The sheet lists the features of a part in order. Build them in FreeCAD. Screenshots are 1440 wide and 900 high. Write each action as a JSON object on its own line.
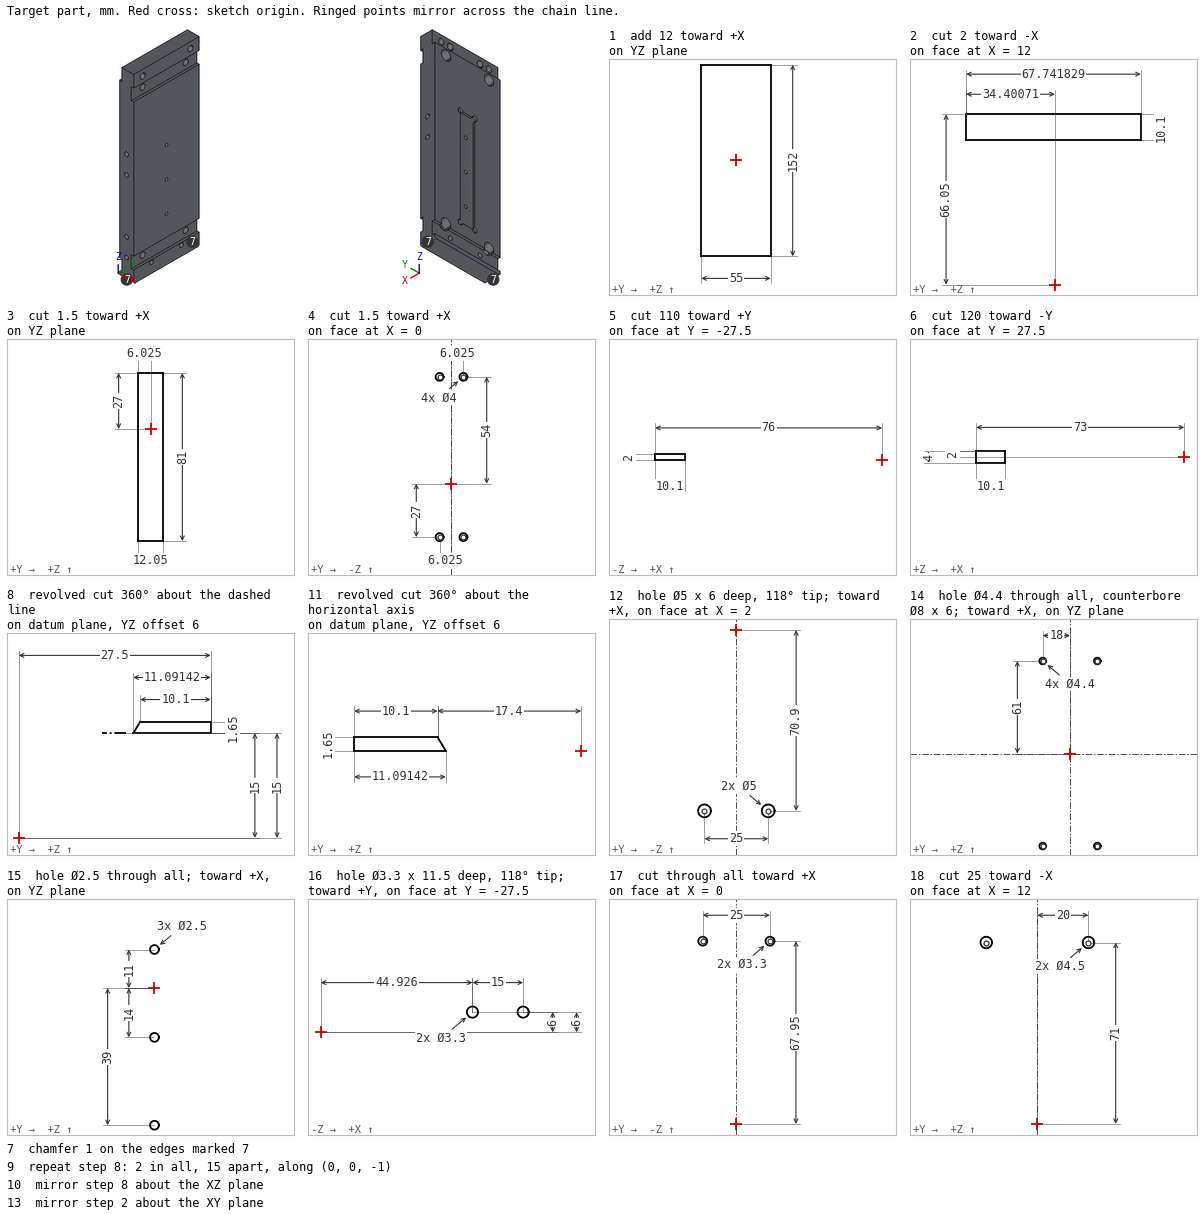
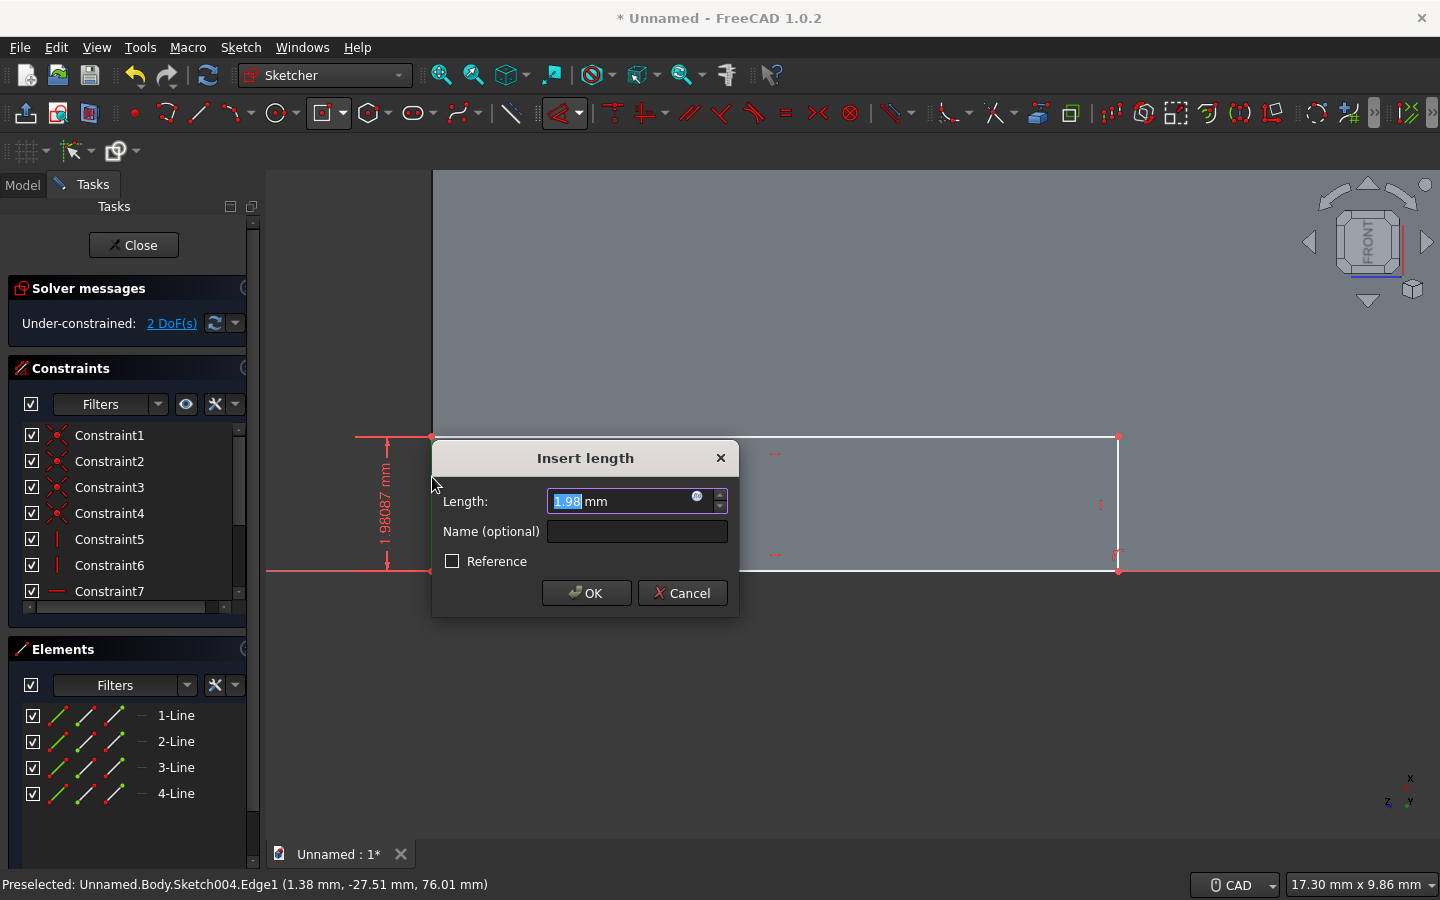
{"action": "type", "text": "2"}
{"action": "key", "text": "Return"}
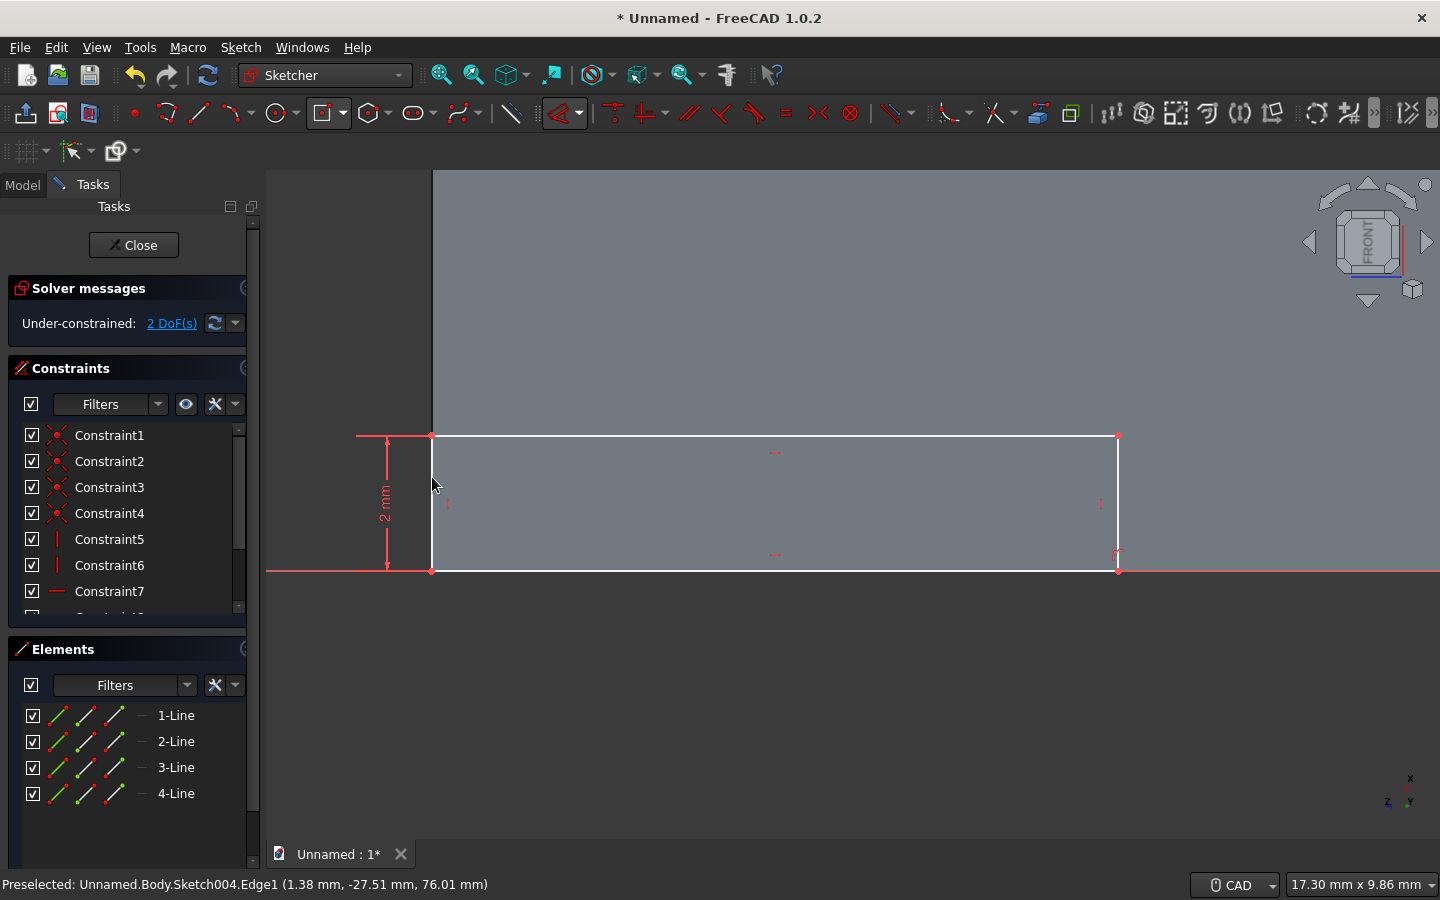
{"action": "left_click", "coordinate": [432, 436]}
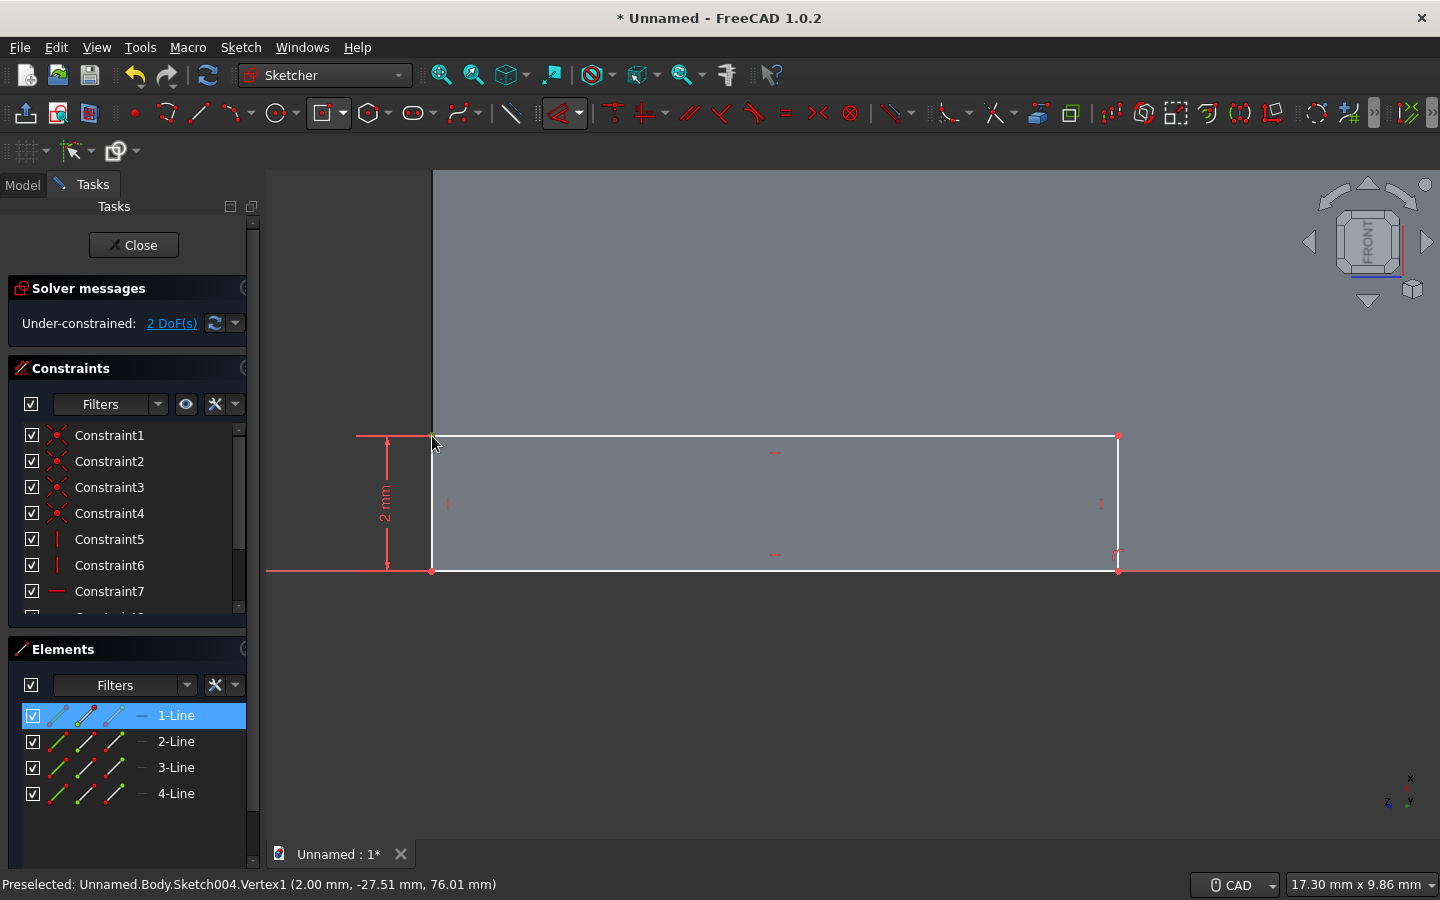
{"action": "left_click", "coordinate": [582, 114]}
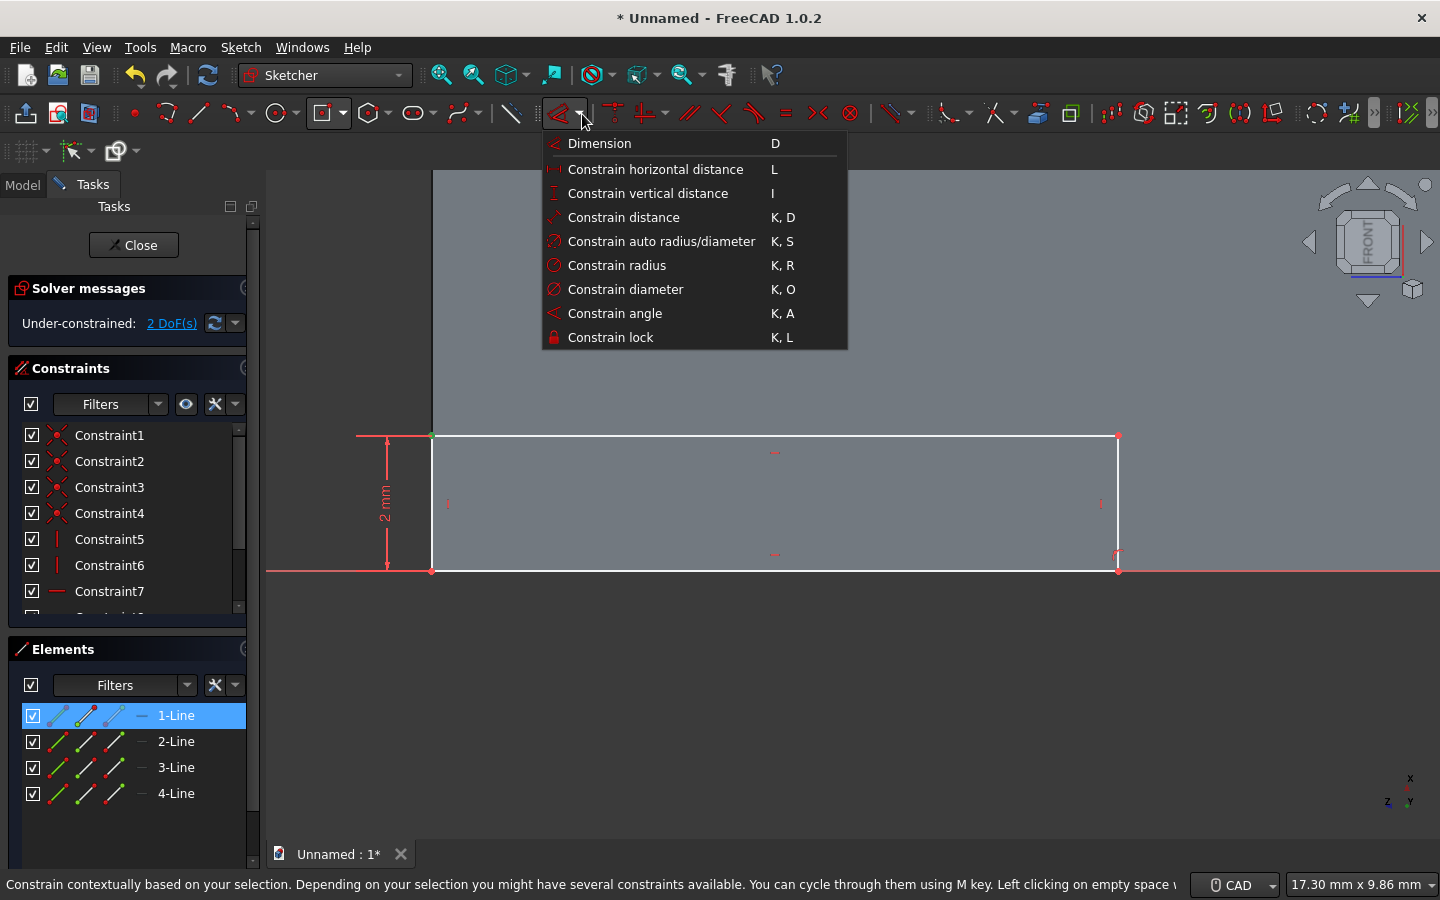
{"action": "left_click", "coordinate": [695, 169]}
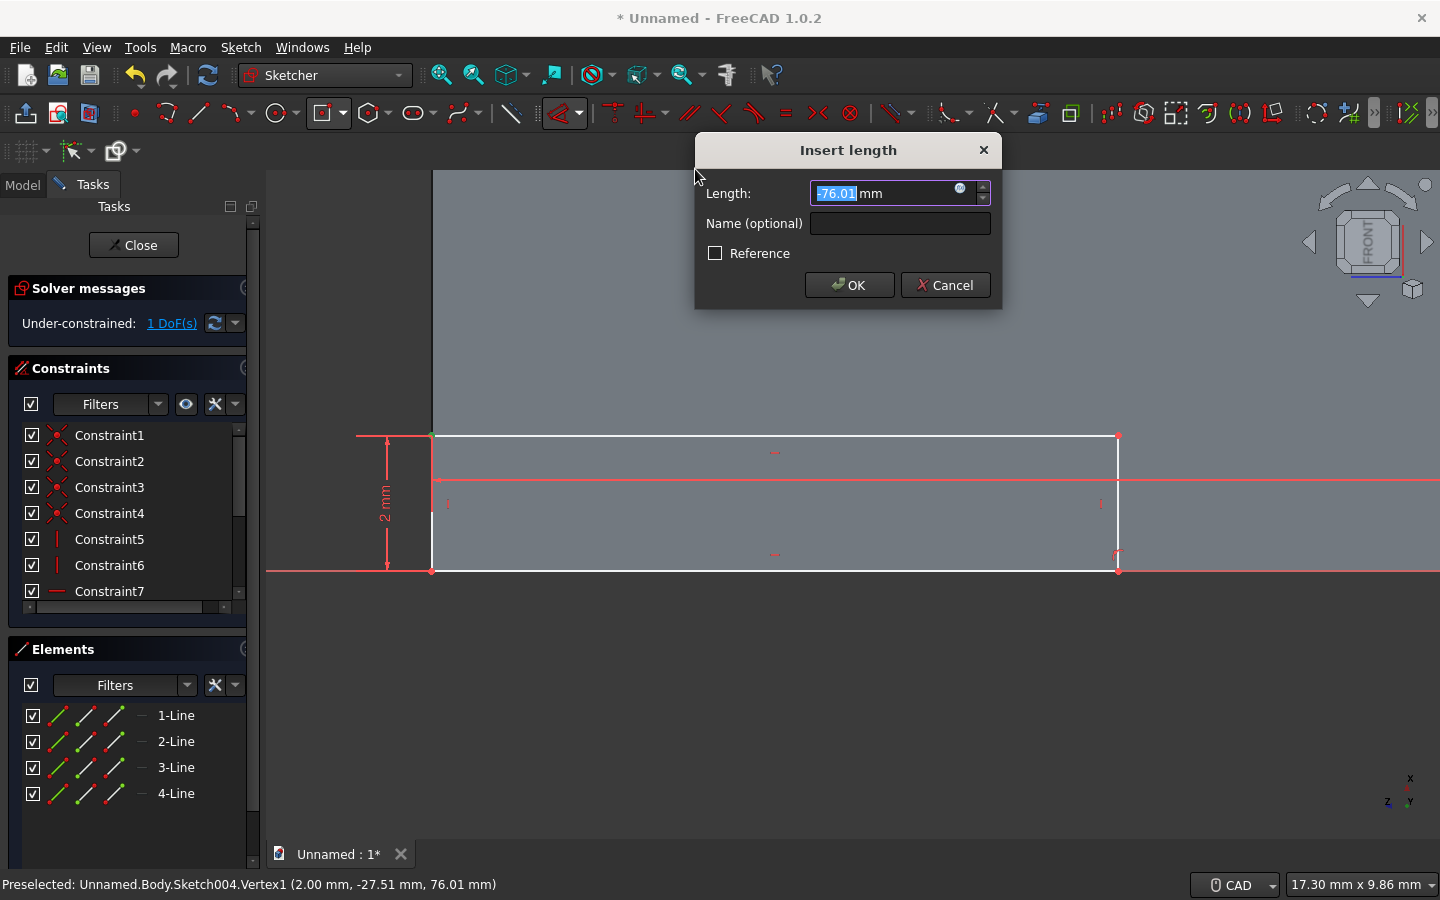
{"action": "type", "text": "-76"}
{"action": "key", "text": "Return"}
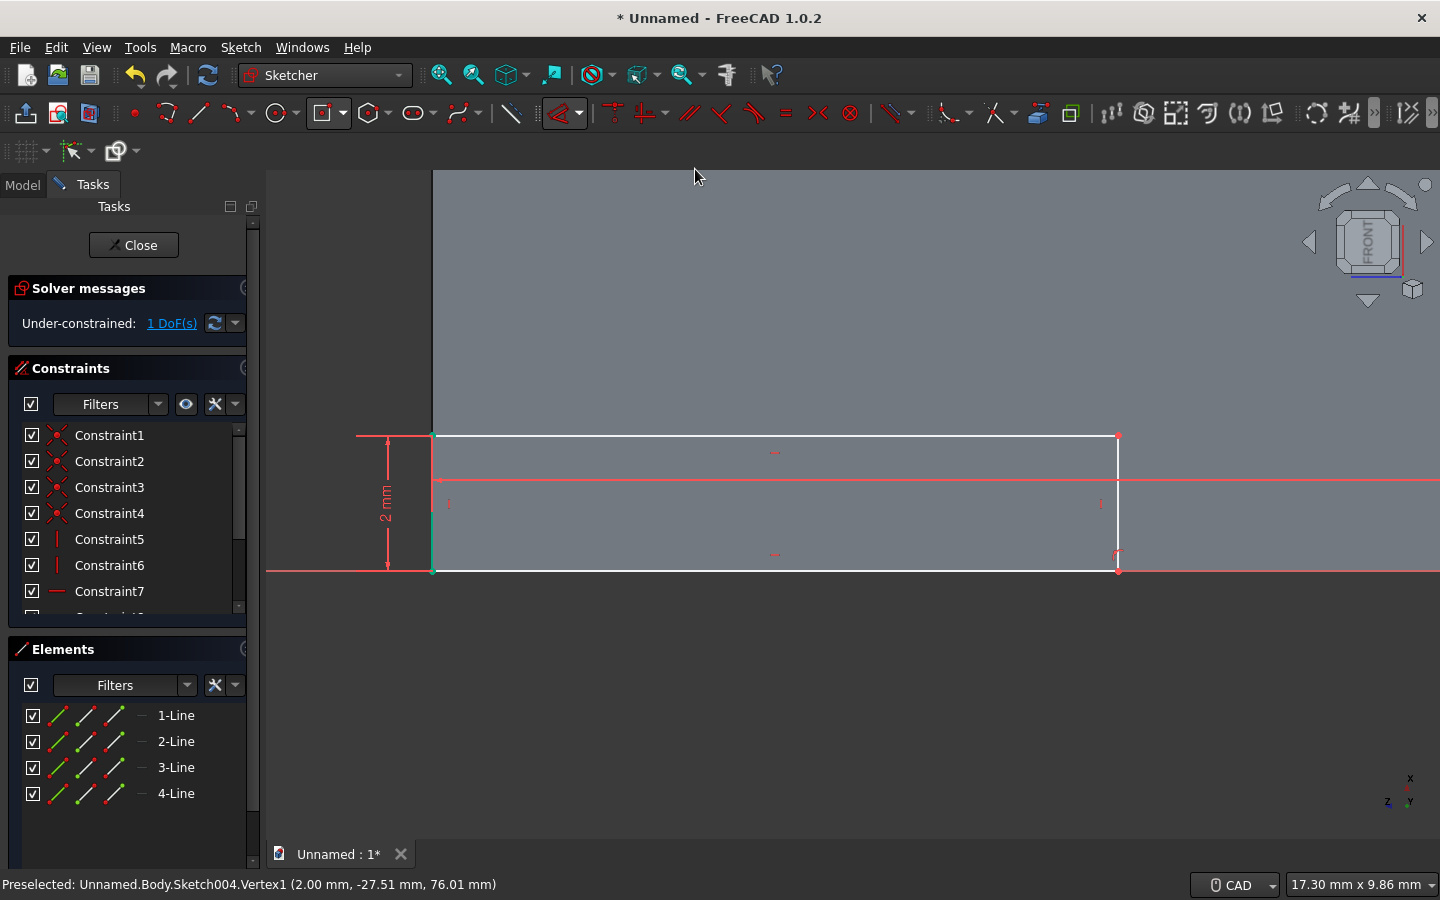
{"action": "left_click", "coordinate": [638, 571]}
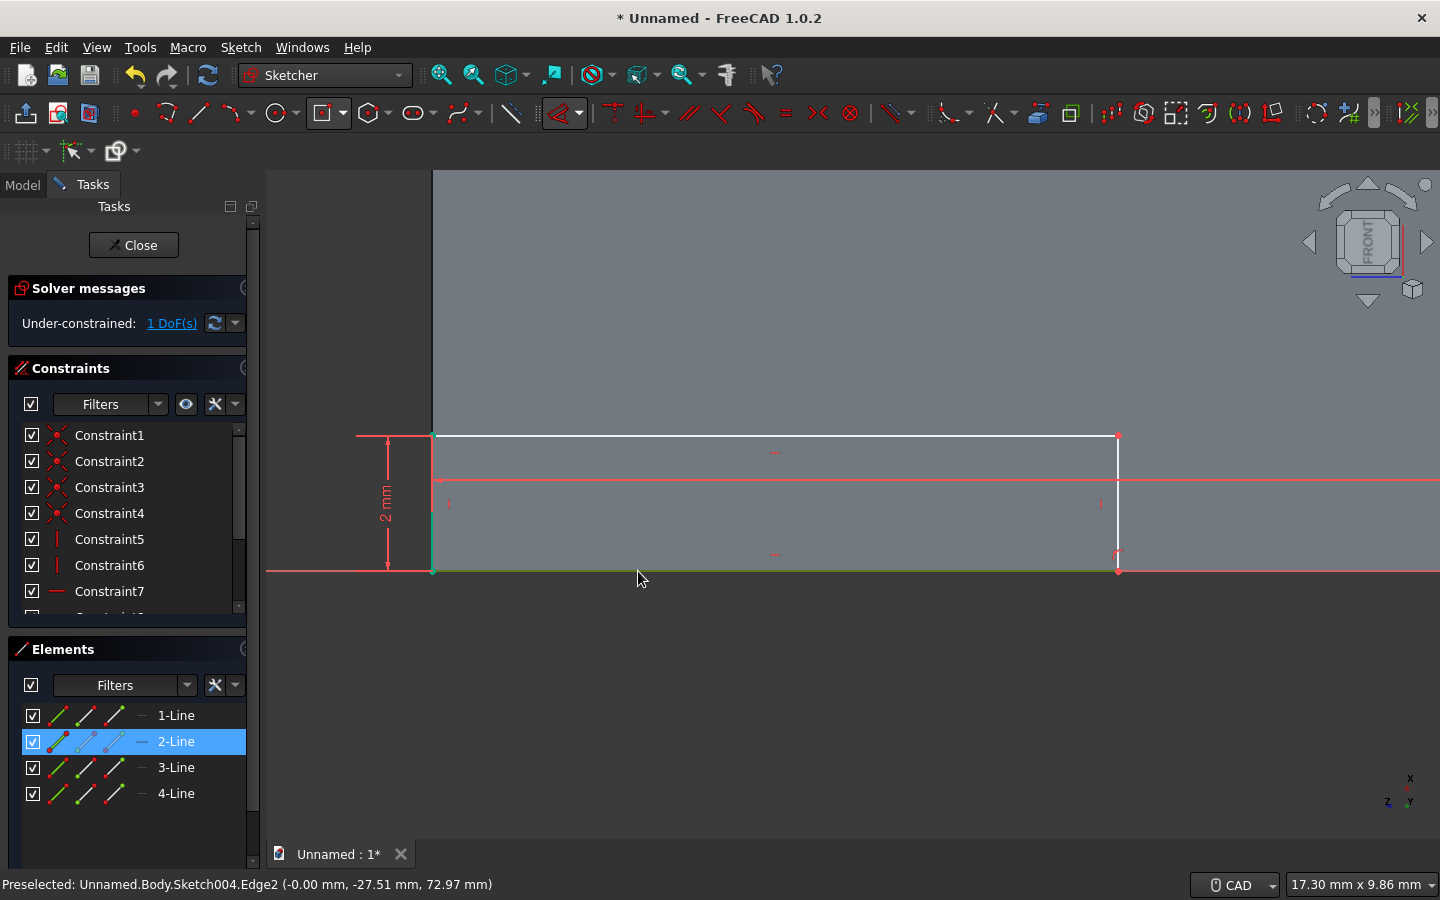
{"action": "left_click", "coordinate": [582, 114]}